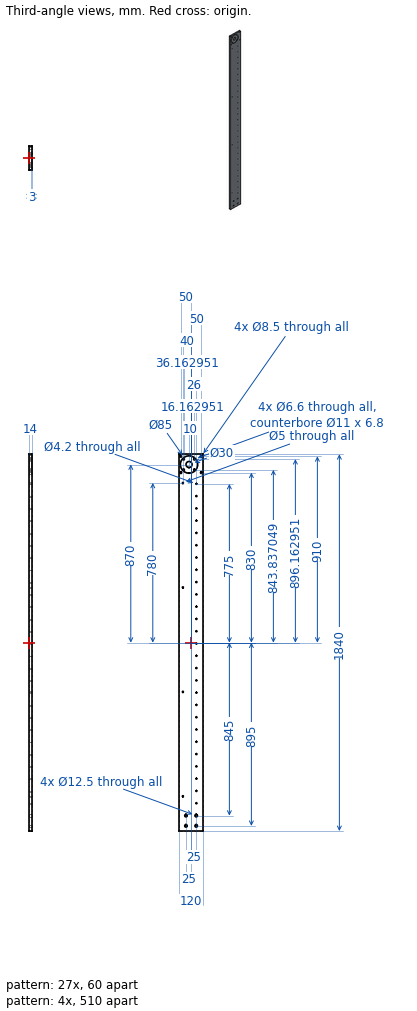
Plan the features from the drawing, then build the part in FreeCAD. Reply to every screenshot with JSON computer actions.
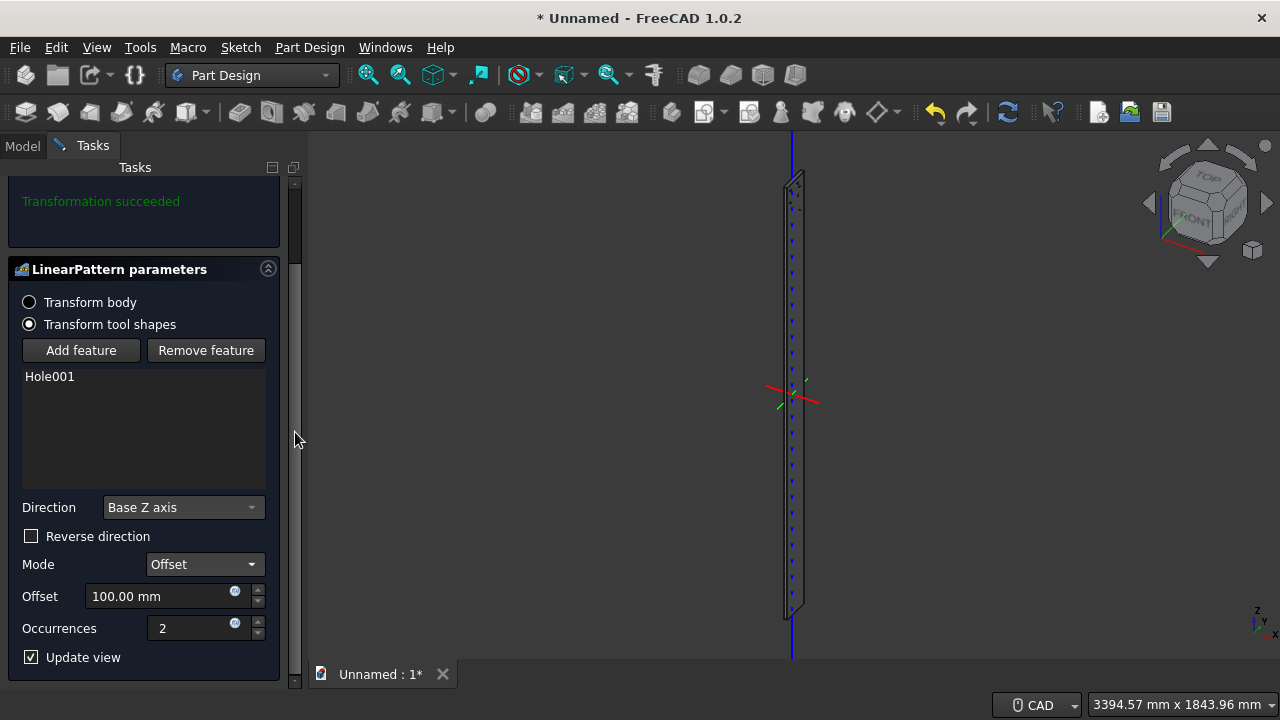
{"action": "triple_click", "coordinate": [168, 596]}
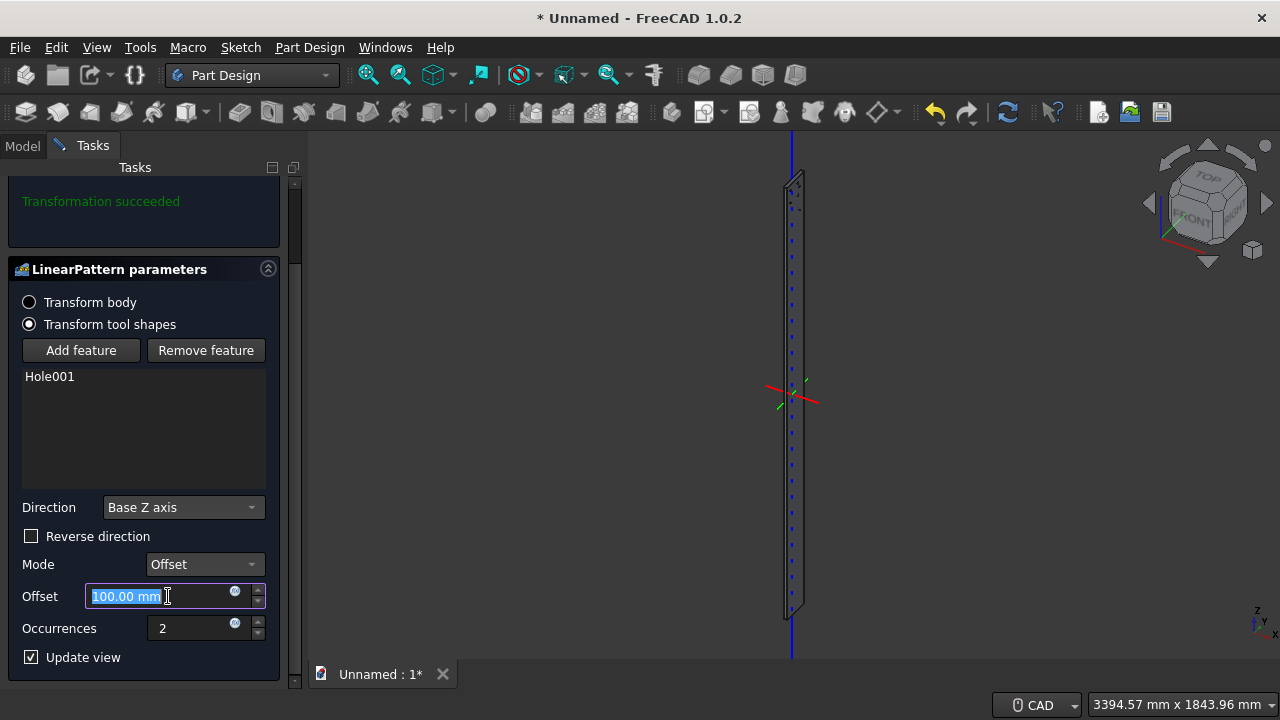
{"action": "type", "text": "60"}
{"action": "key", "text": "Tab"}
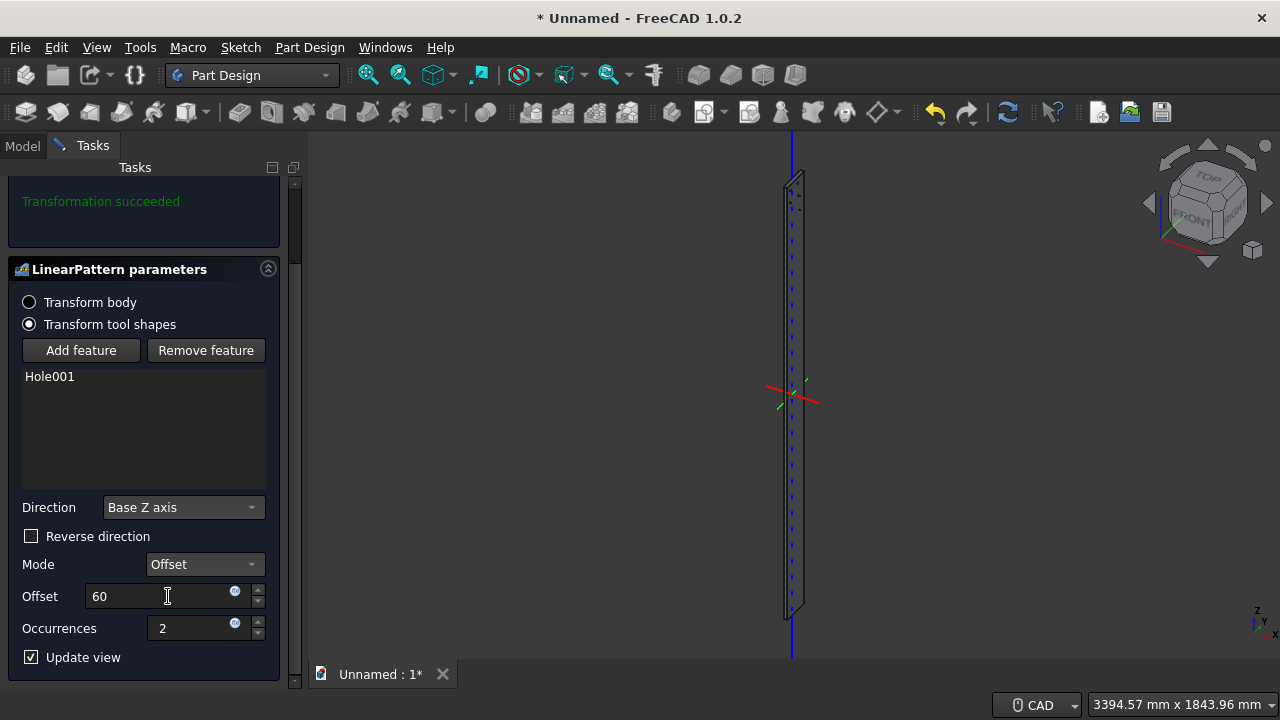
{"action": "triple_click", "coordinate": [198, 628]}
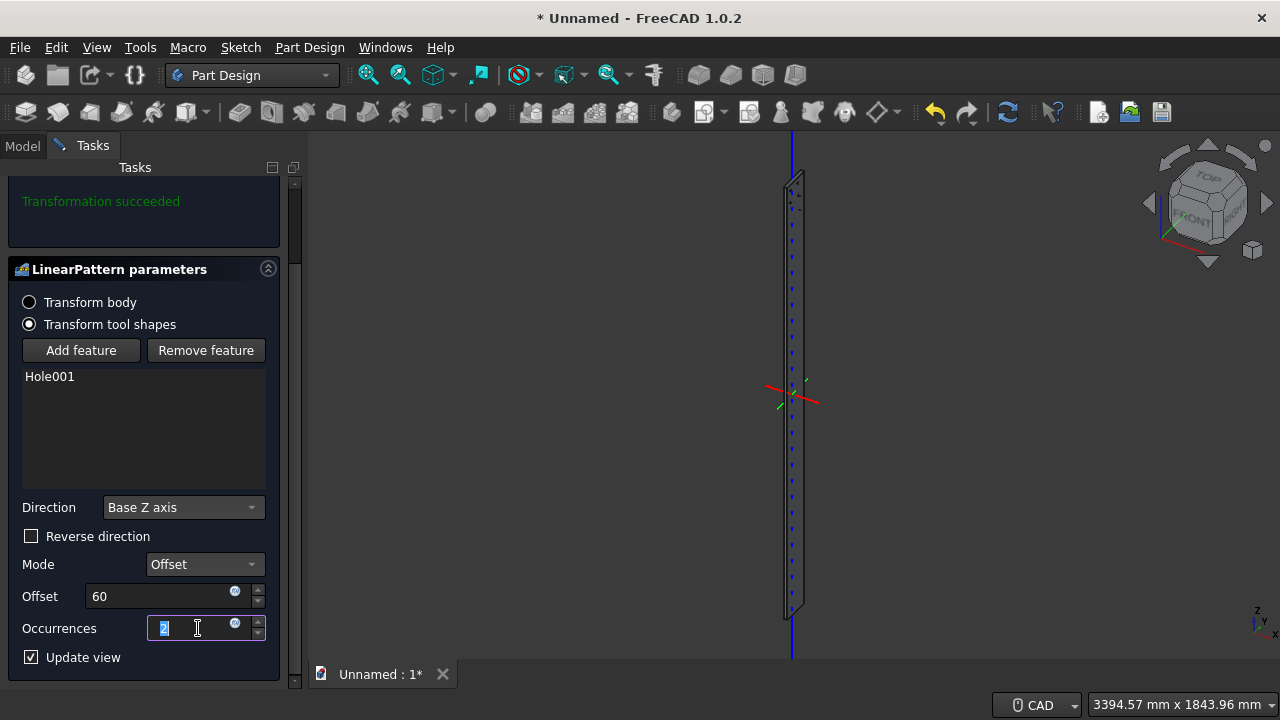
{"action": "type", "text": "27"}
{"action": "key", "text": "Tab"}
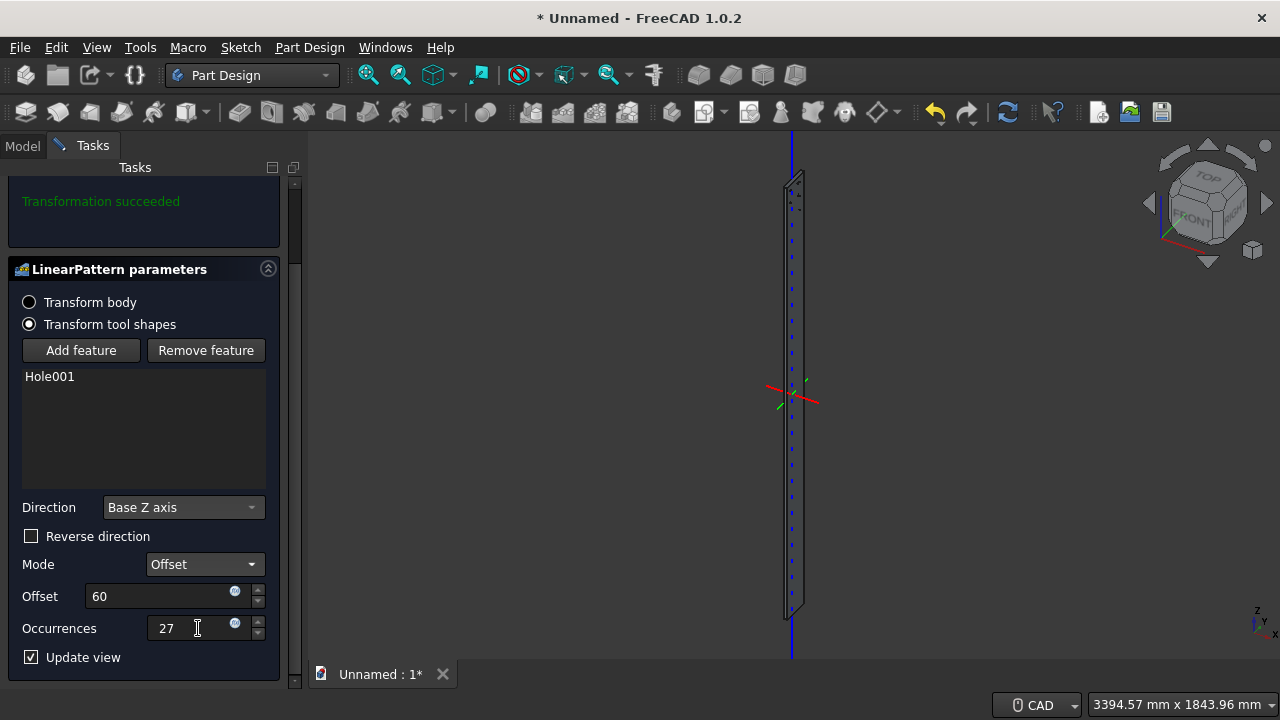
{"action": "left_click", "coordinate": [30, 536]}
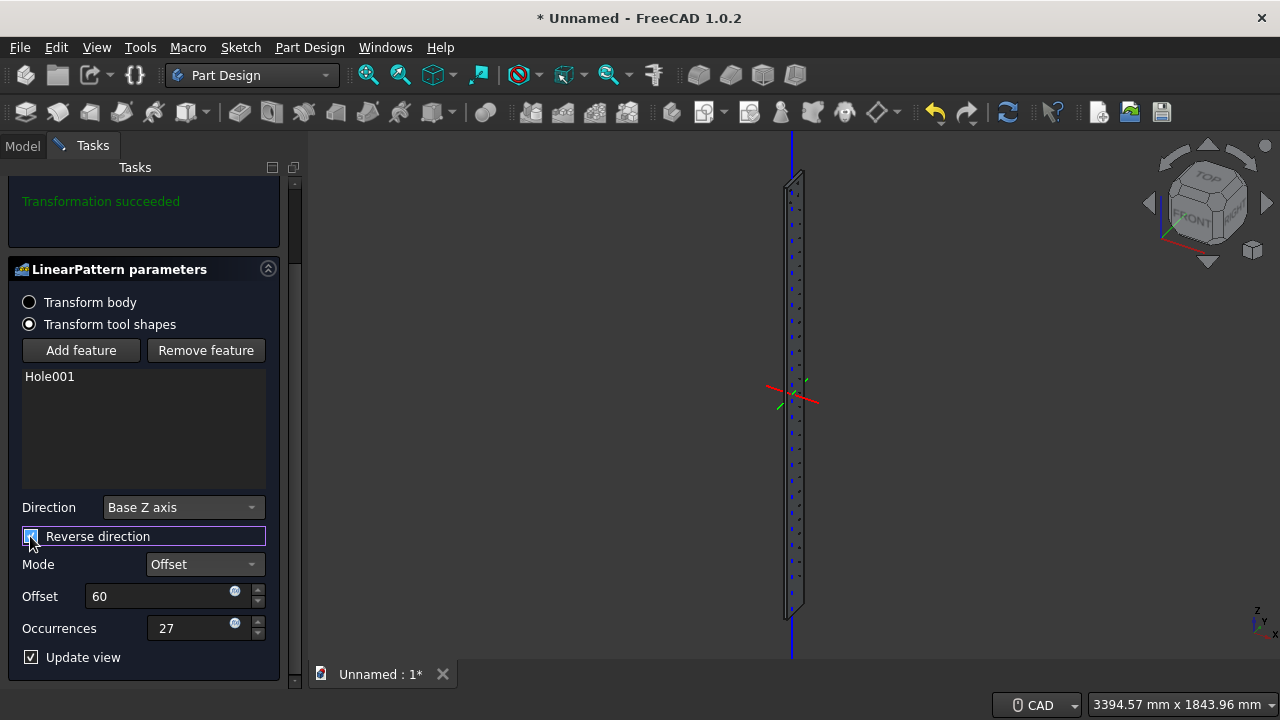
{"action": "scroll", "coordinate": [295, 432], "scroll_direction": "up", "scroll_amount": 3}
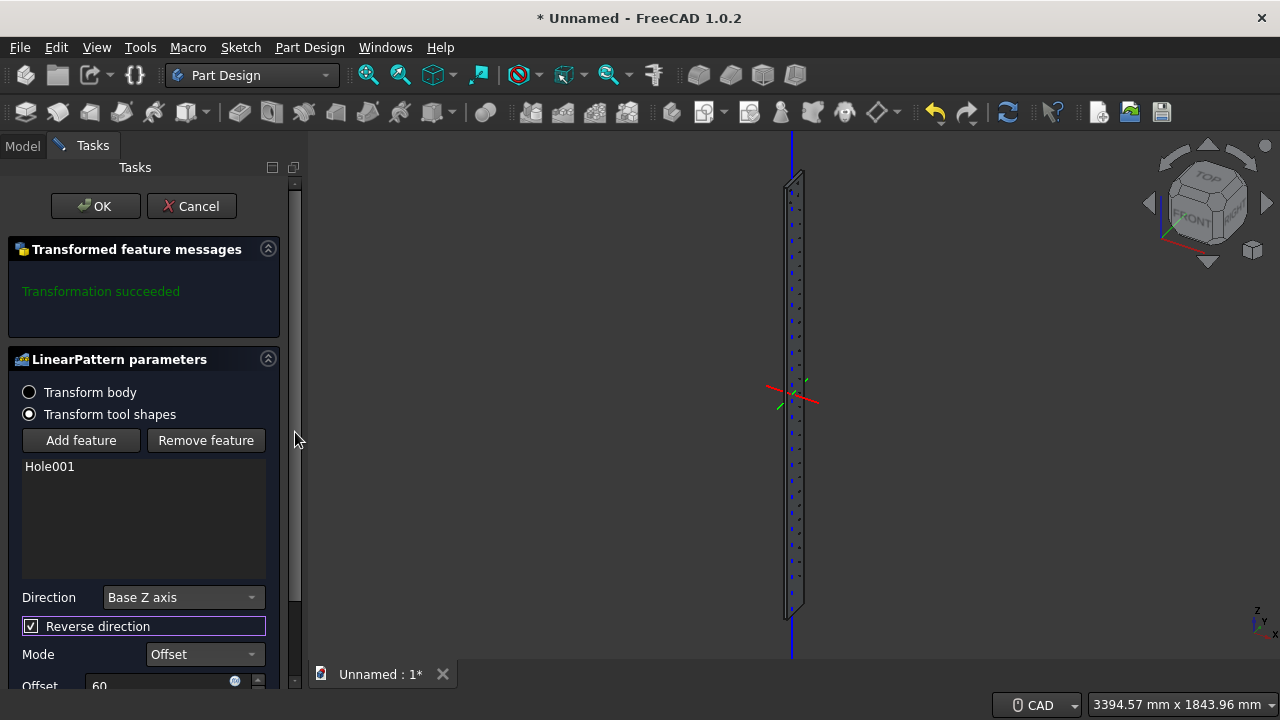
{"action": "left_click", "coordinate": [96, 206]}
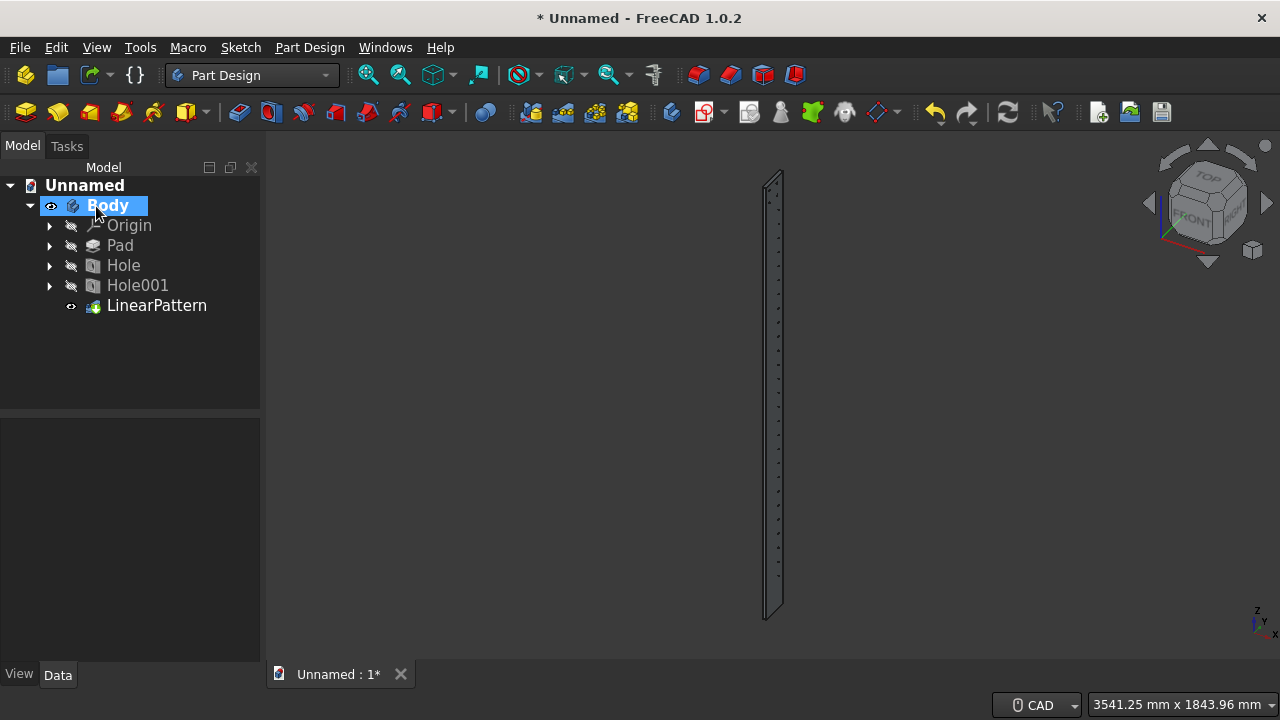
{"action": "left_click", "coordinate": [775, 333]}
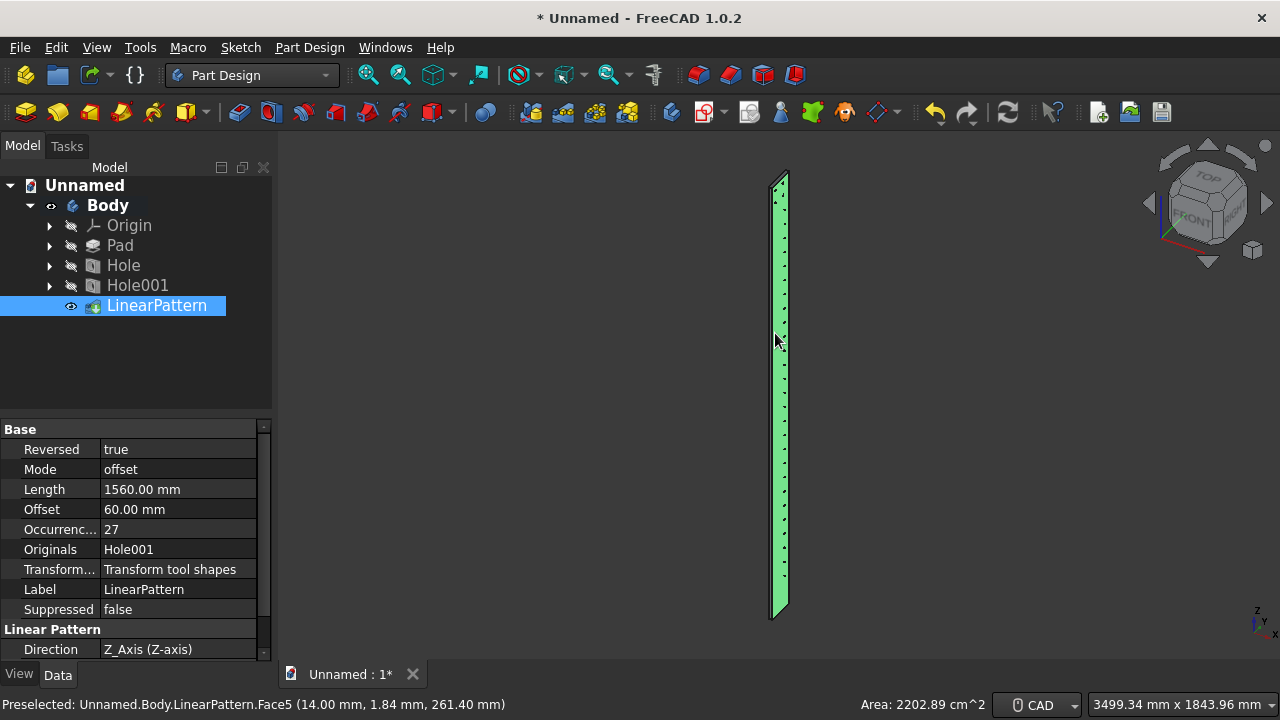
{"action": "left_click", "coordinate": [704, 112]}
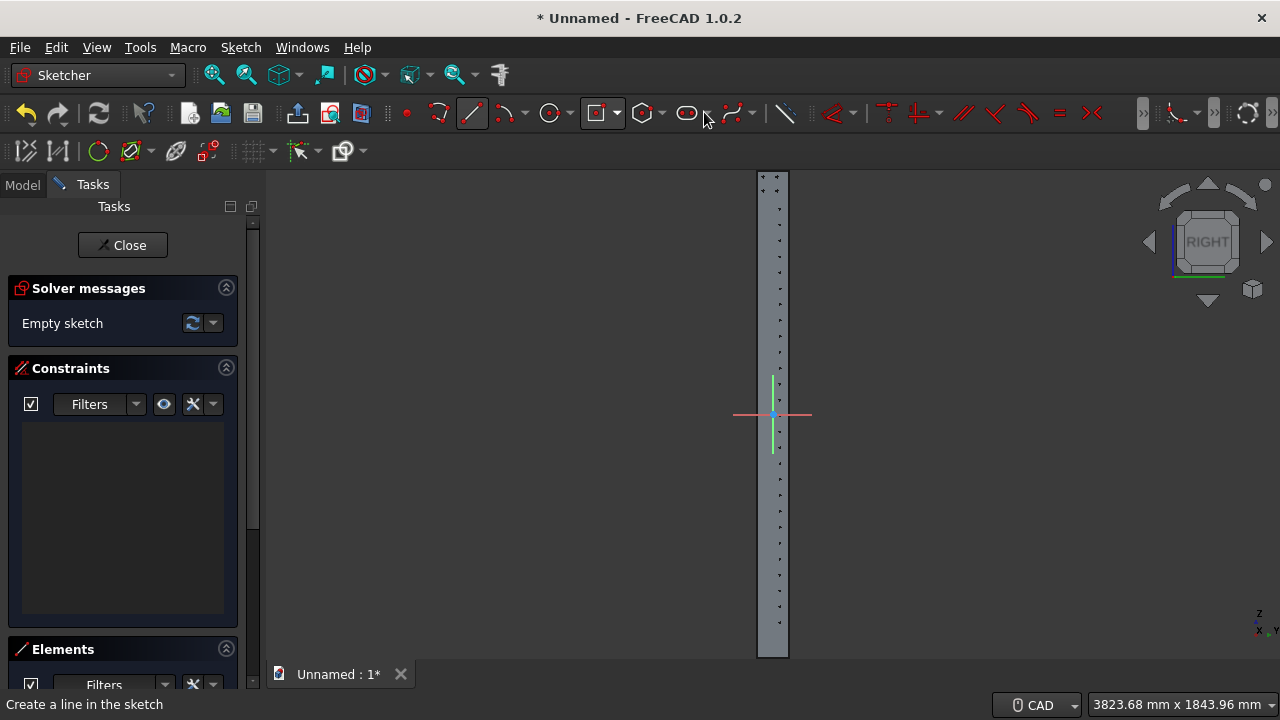
{"action": "scroll", "coordinate": [704, 414], "scroll_direction": "down", "scroll_amount": 5}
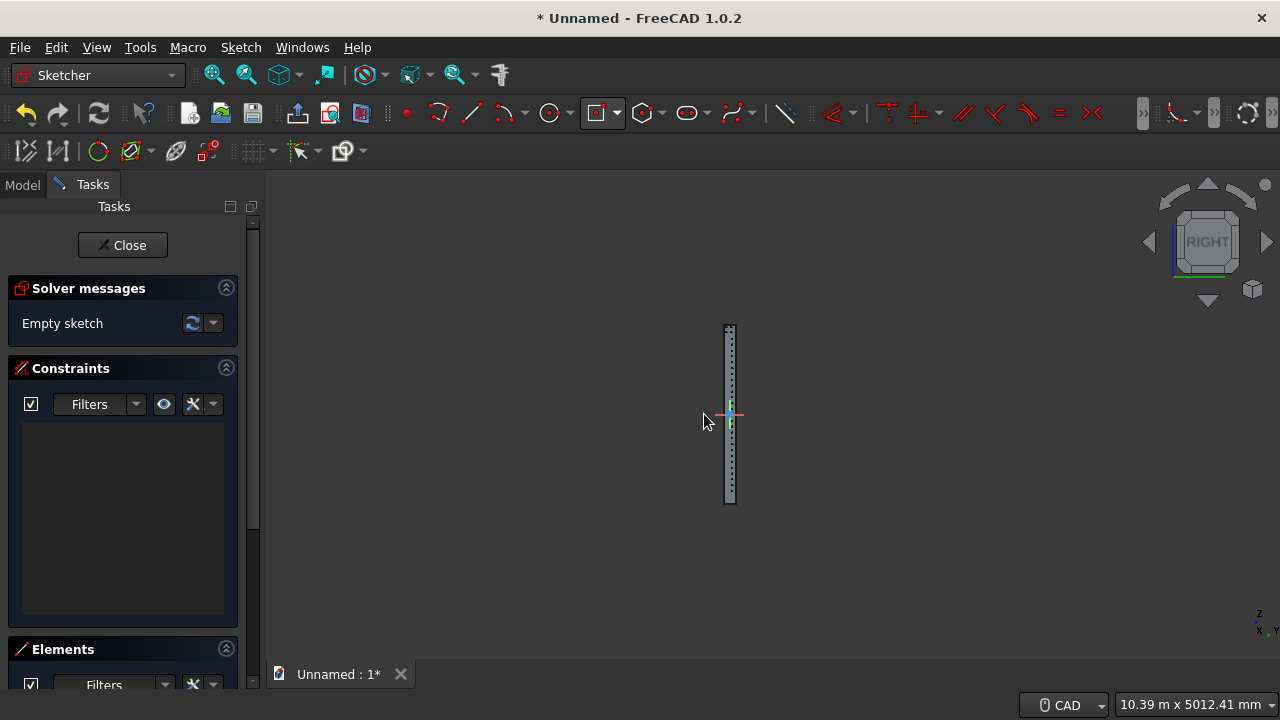
{"action": "scroll", "coordinate": [731, 504], "scroll_direction": "up", "scroll_amount": 15}